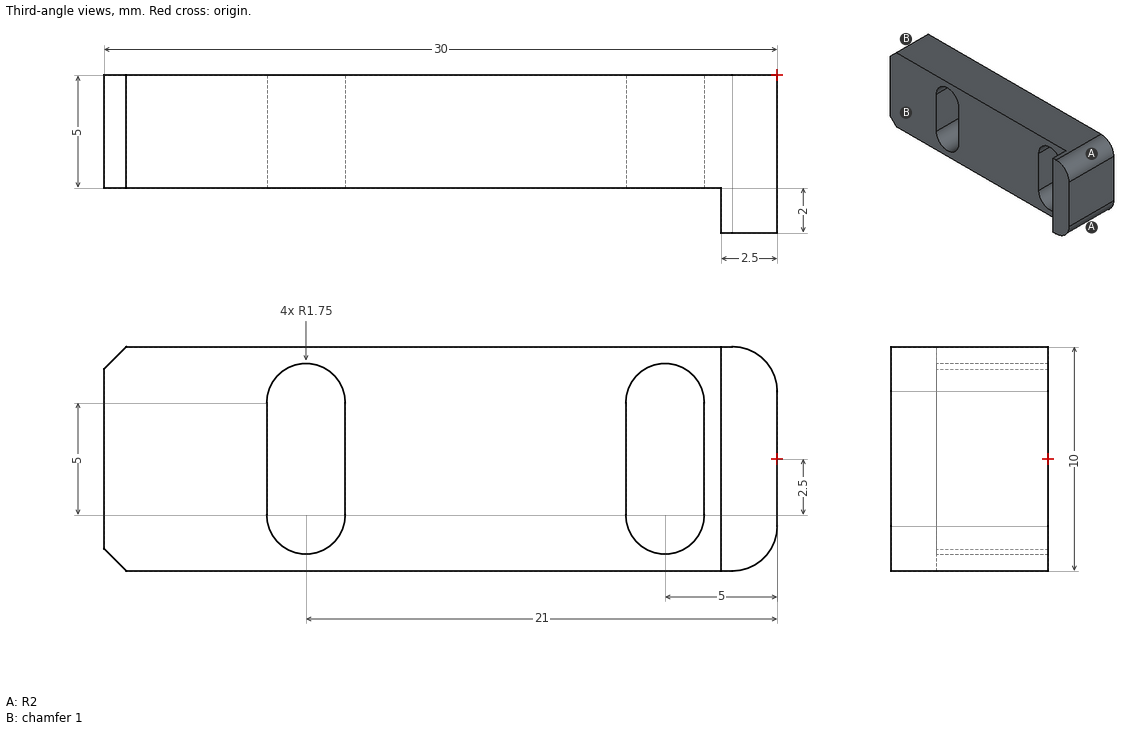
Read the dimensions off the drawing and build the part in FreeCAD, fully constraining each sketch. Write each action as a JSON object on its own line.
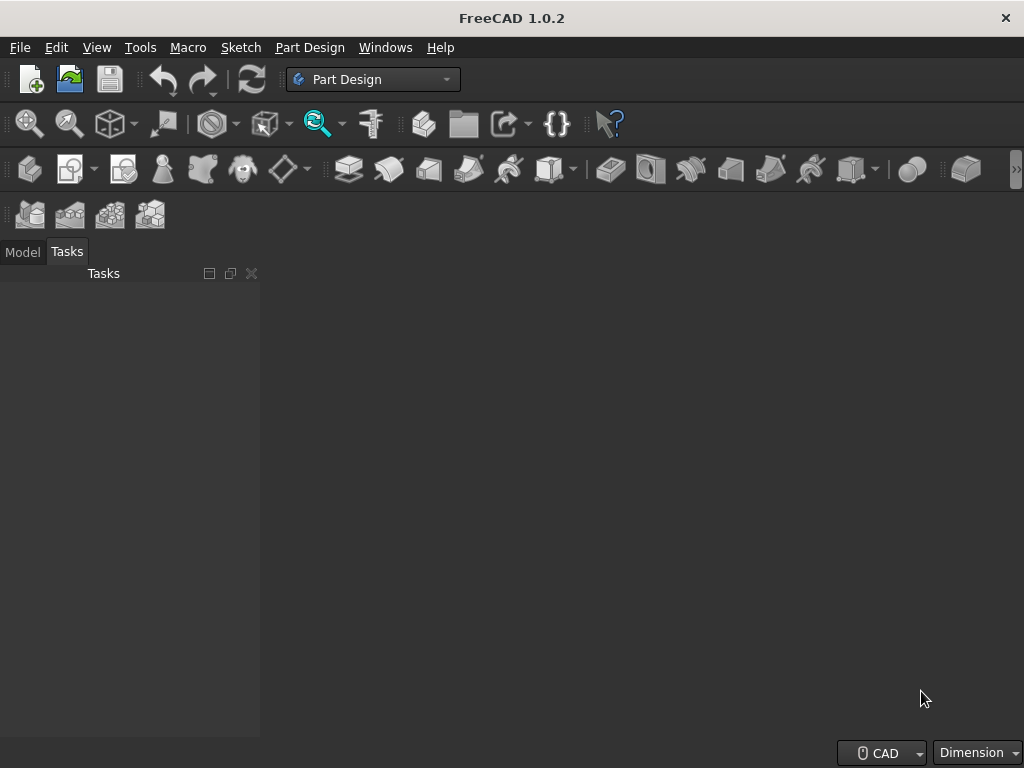
{"action": "left_click", "coordinate": [30, 80]}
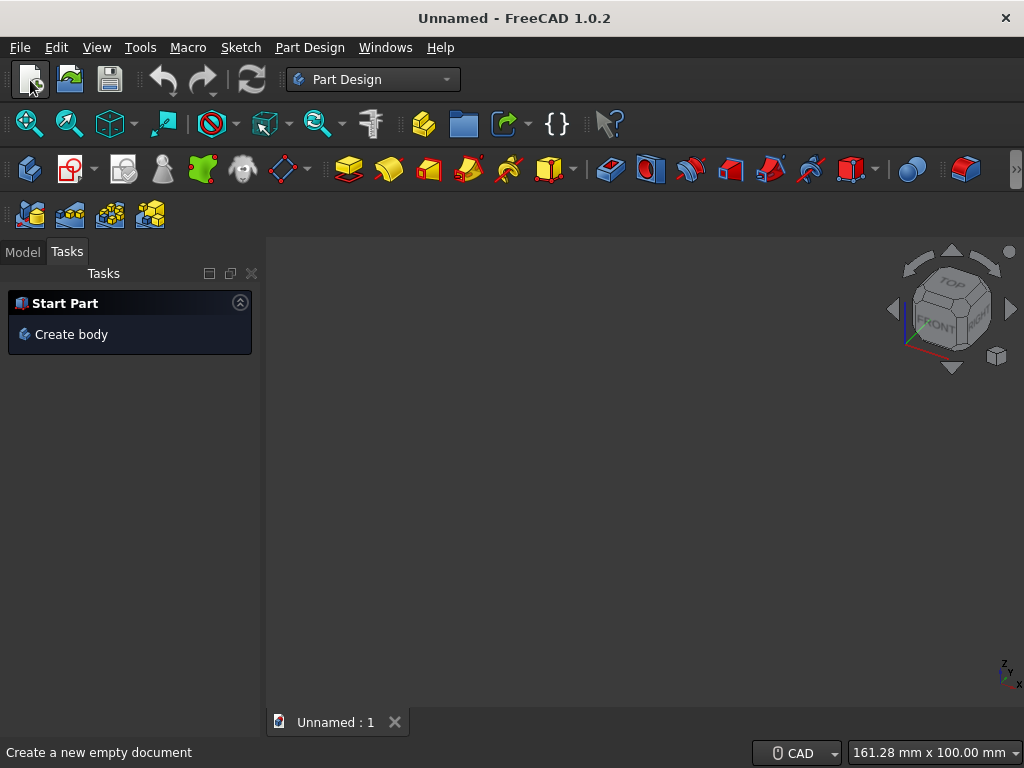
{"action": "left_click", "coordinate": [70, 170]}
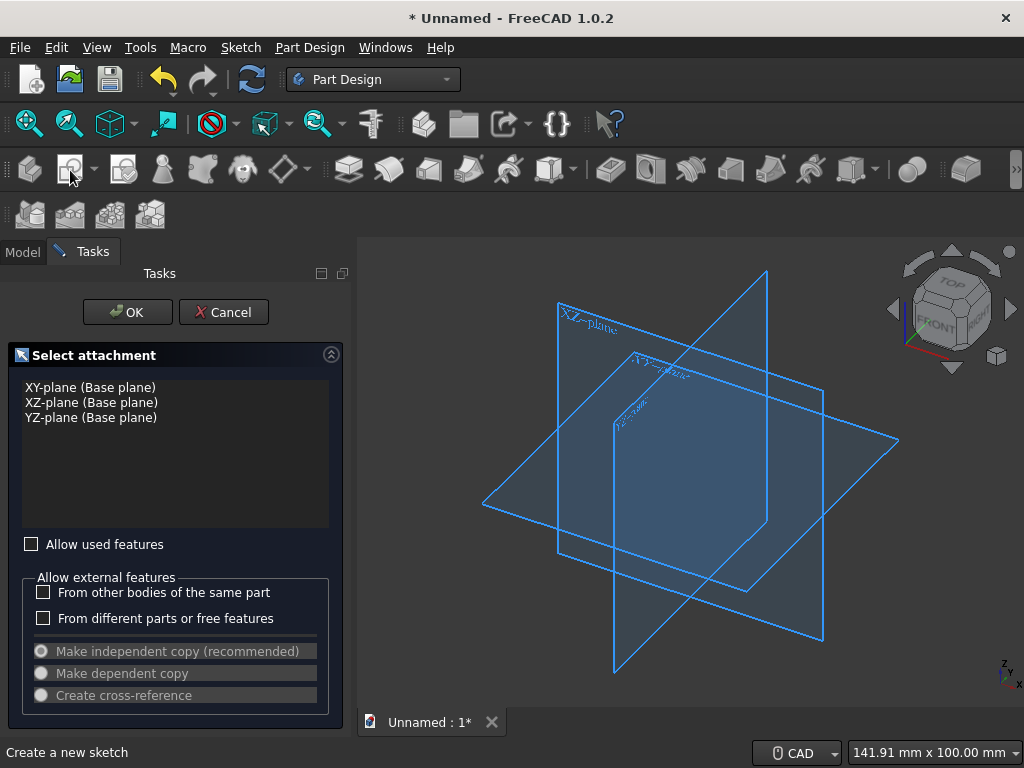
{"action": "left_click", "coordinate": [82, 388]}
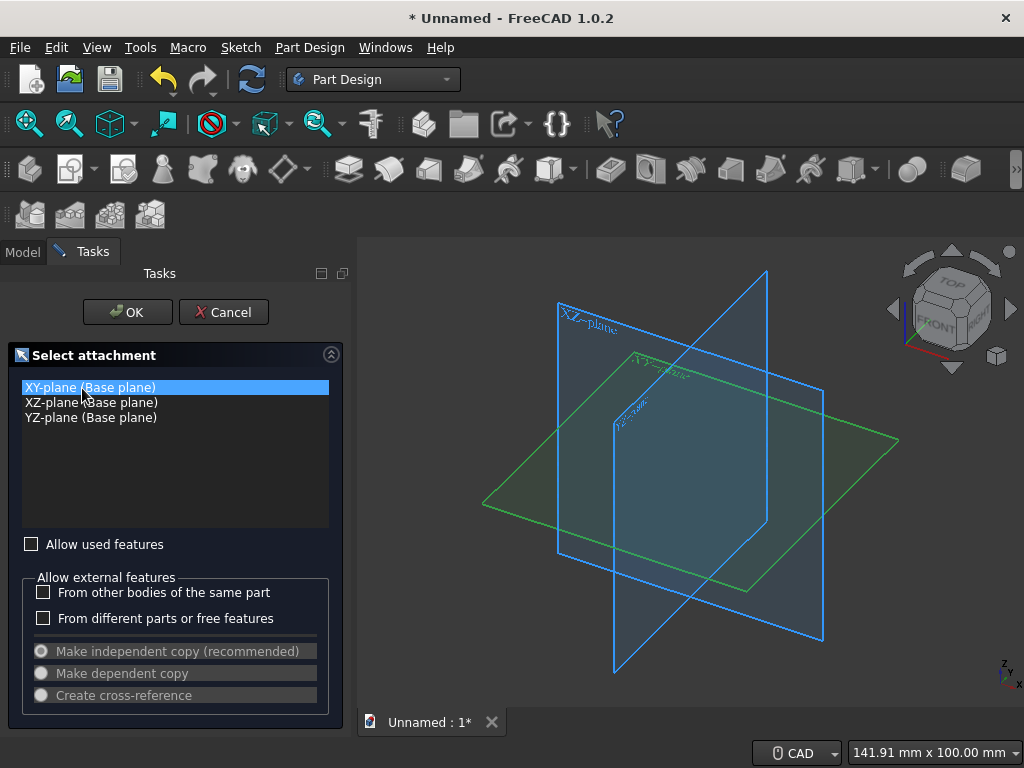
{"action": "left_click", "coordinate": [128, 312]}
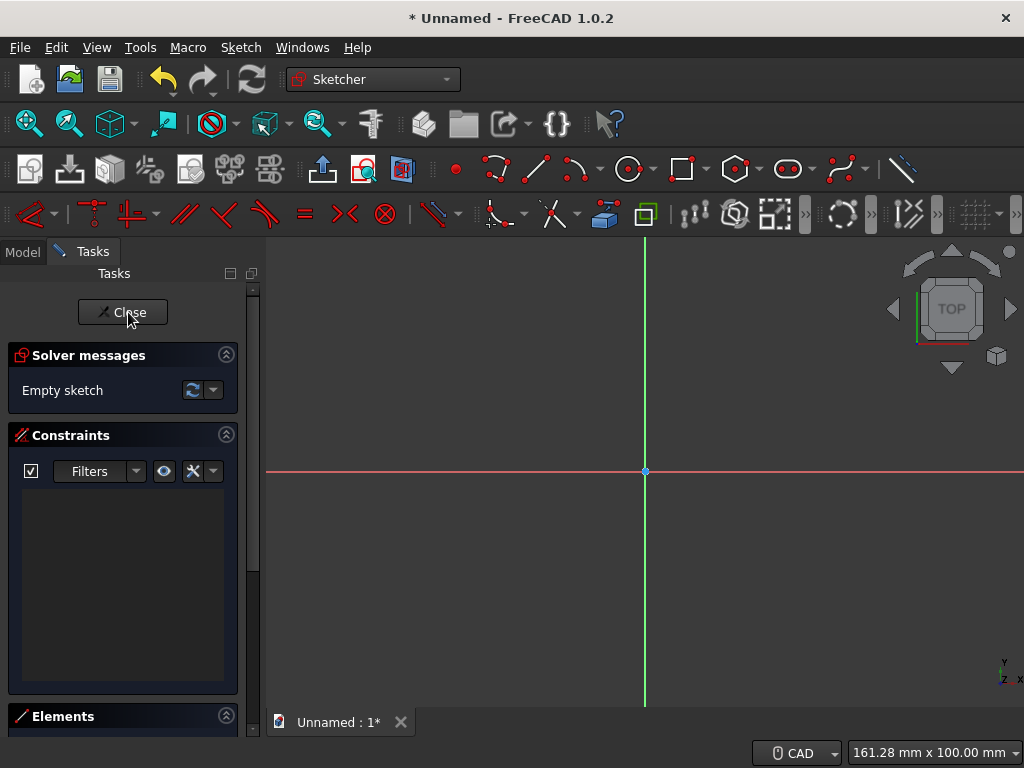
{"action": "scroll", "coordinate": [573, 498], "scroll_direction": "up", "scroll_amount": 5}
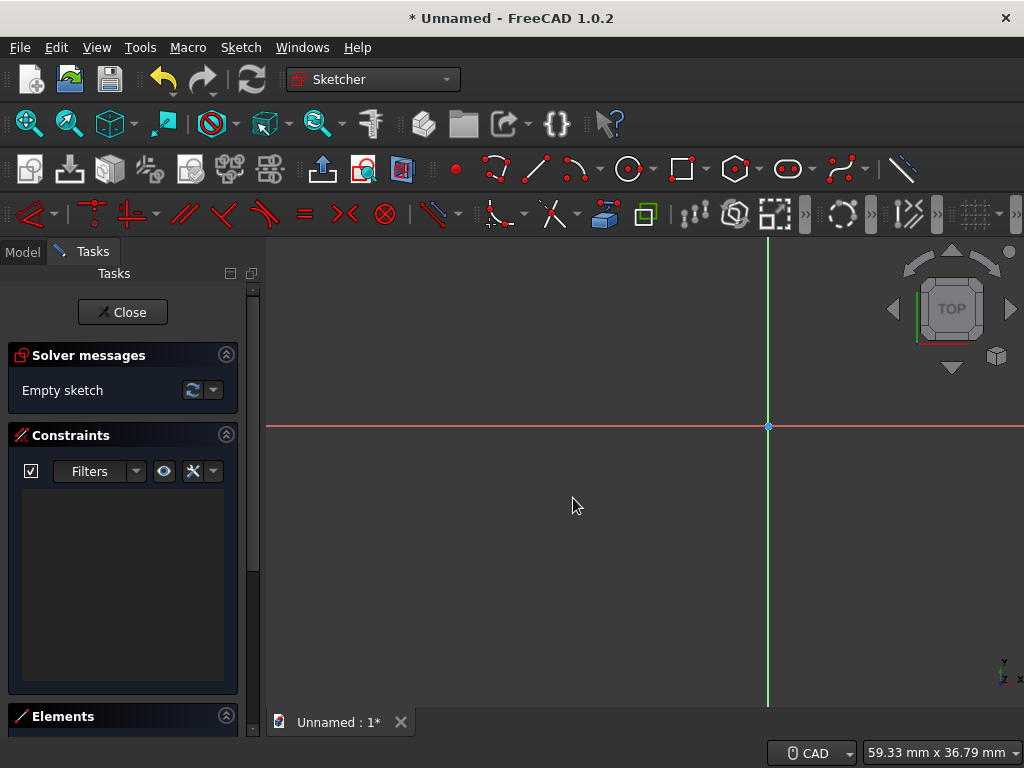
{"action": "left_click", "coordinate": [496, 170]}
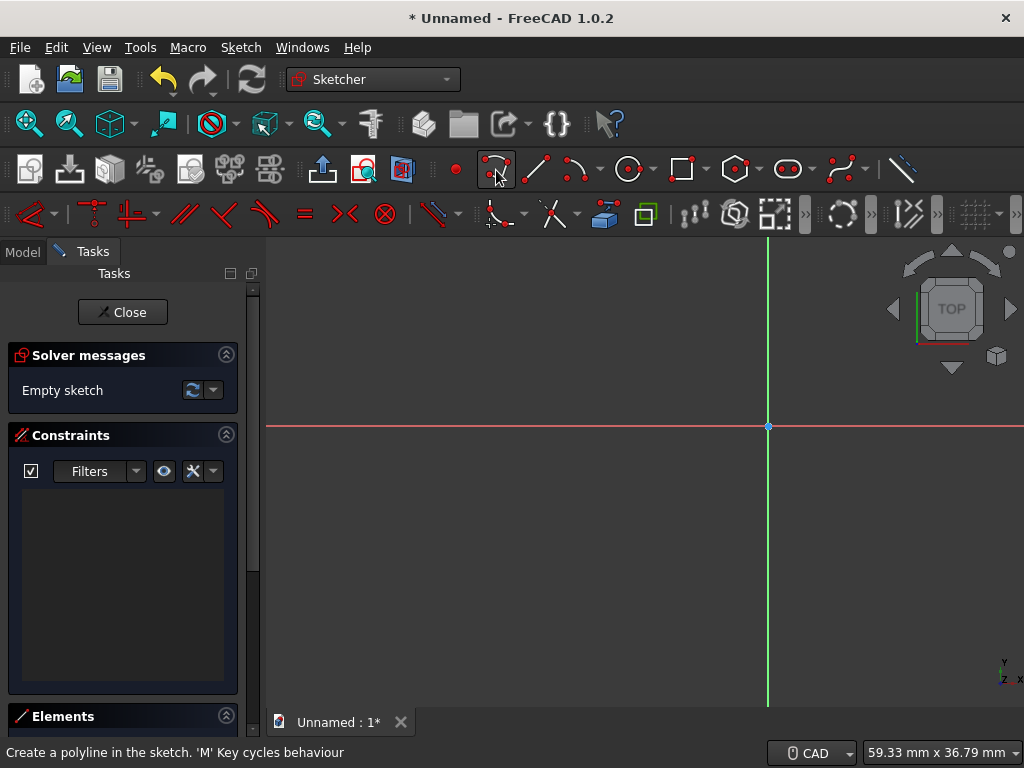
{"action": "left_click", "coordinate": [768, 426]}
{"action": "left_click", "coordinate": [385, 435]}
{"action": "left_click", "coordinate": [385, 490]}
{"action": "left_click", "coordinate": [736, 490]}
{"action": "left_click", "coordinate": [736, 516]}
{"action": "left_click", "coordinate": [759, 516]}
{"action": "left_click", "coordinate": [768, 426]}
{"action": "key", "text": "Escape"}
{"action": "key", "text": "Escape"}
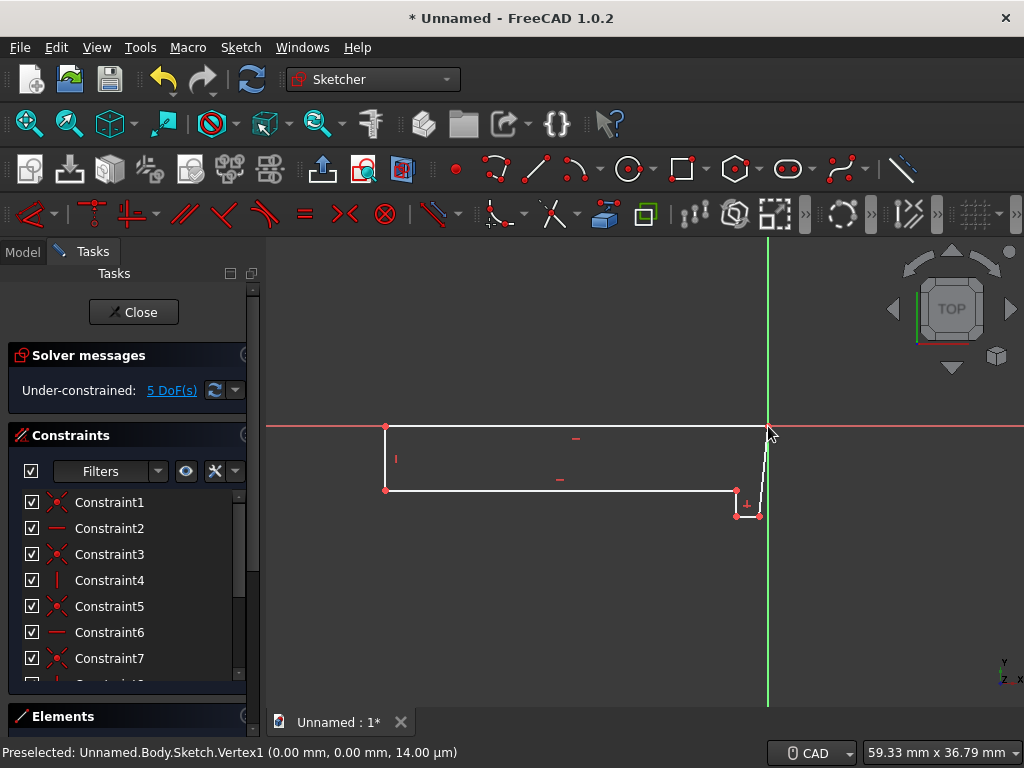
{"action": "left_click", "coordinate": [765, 454]}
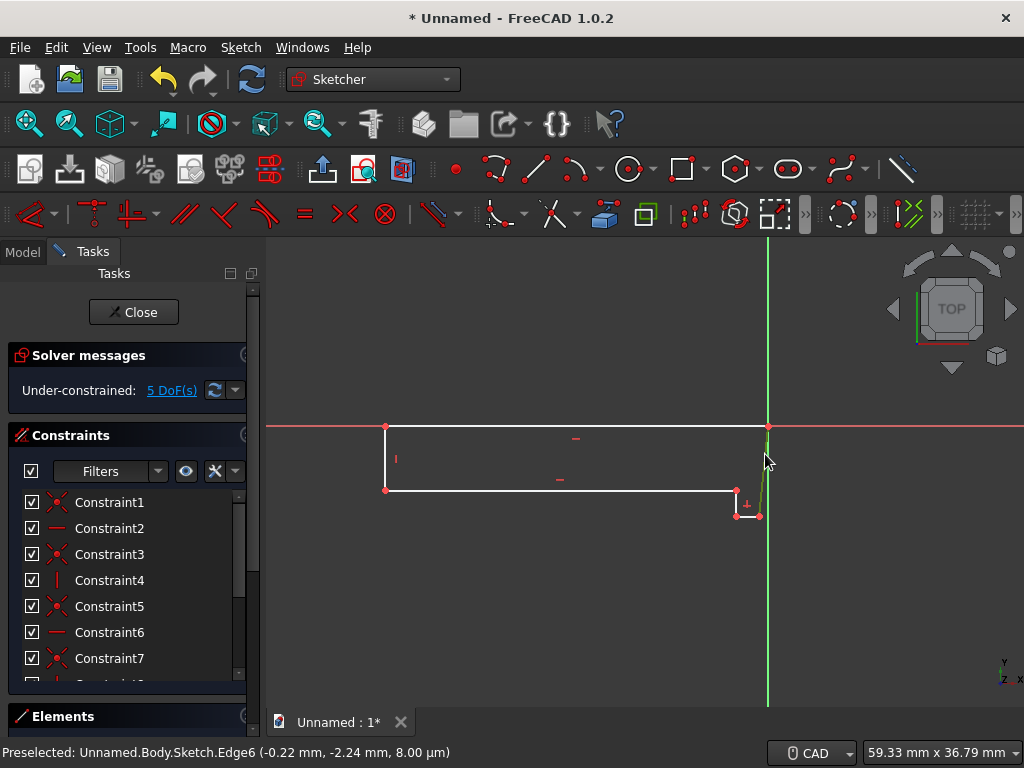
{"action": "left_click", "coordinate": [158, 214]}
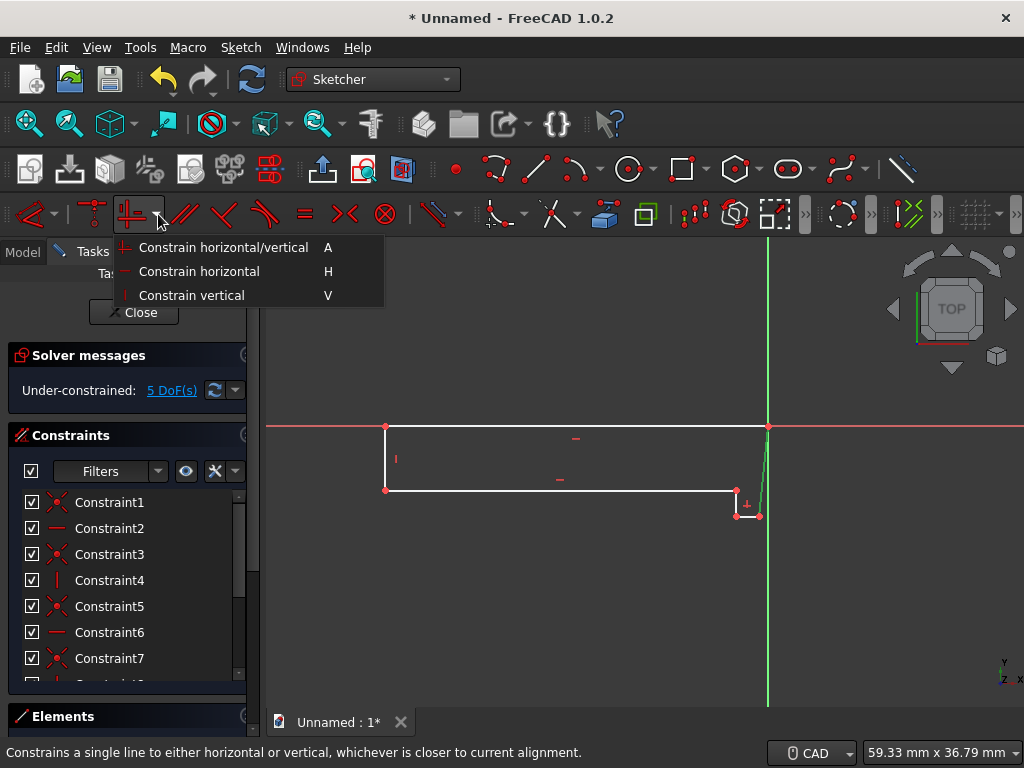
{"action": "left_click", "coordinate": [249, 295]}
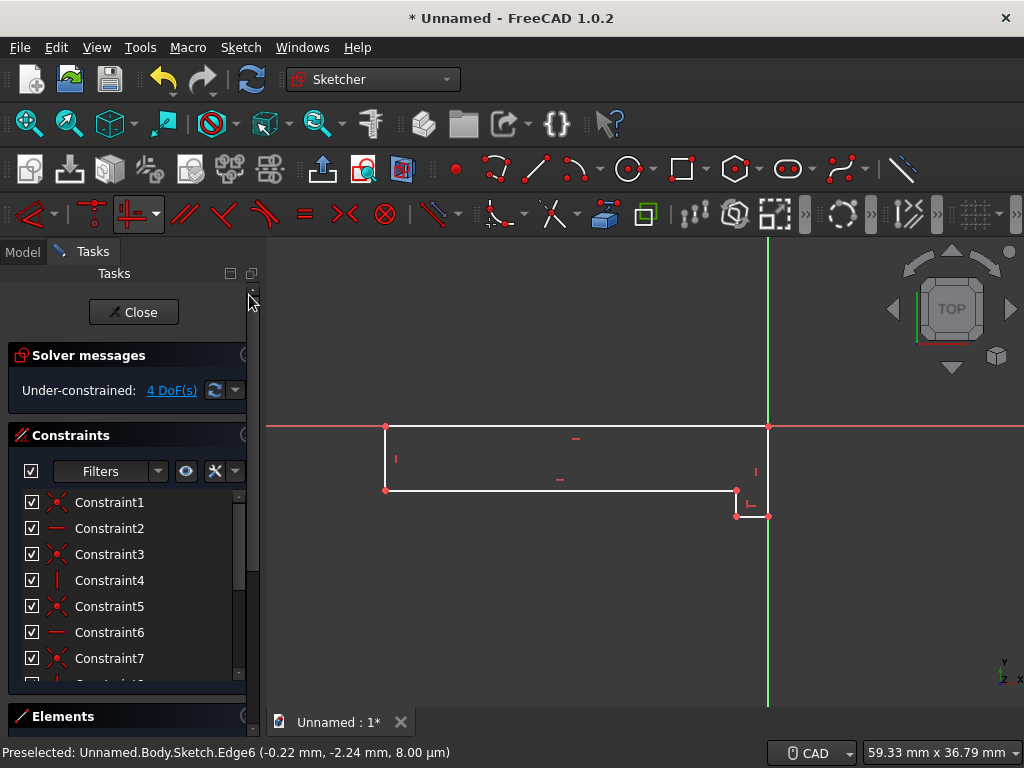
{"action": "left_click", "coordinate": [385, 446]}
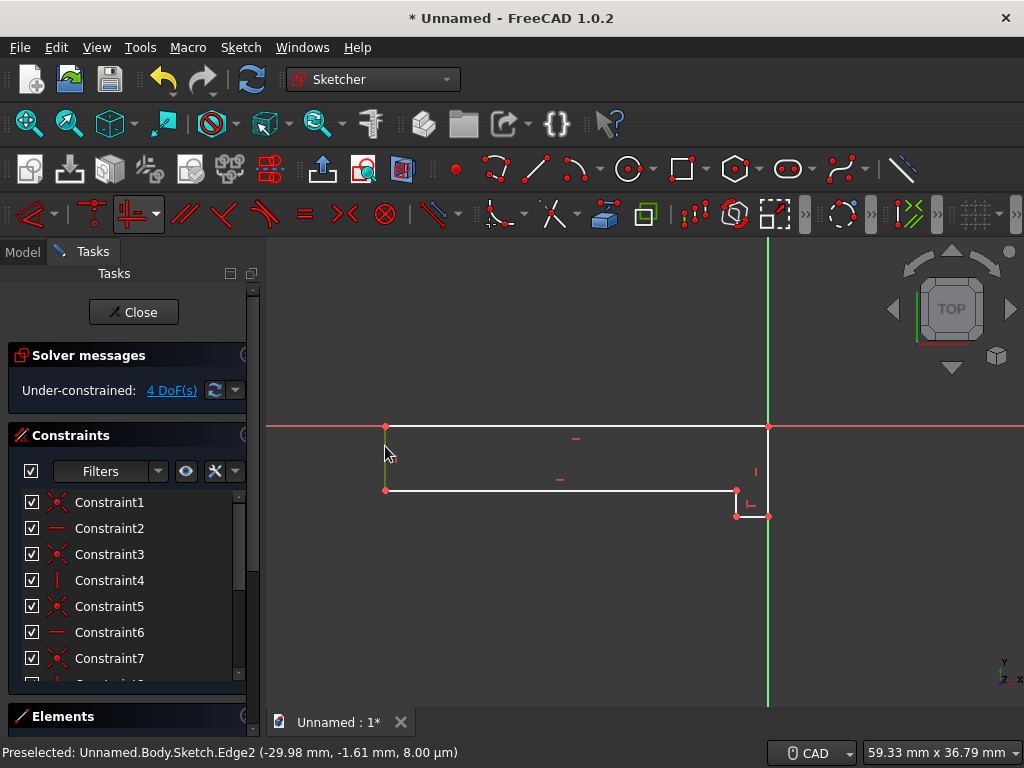
{"action": "key", "text": "i"}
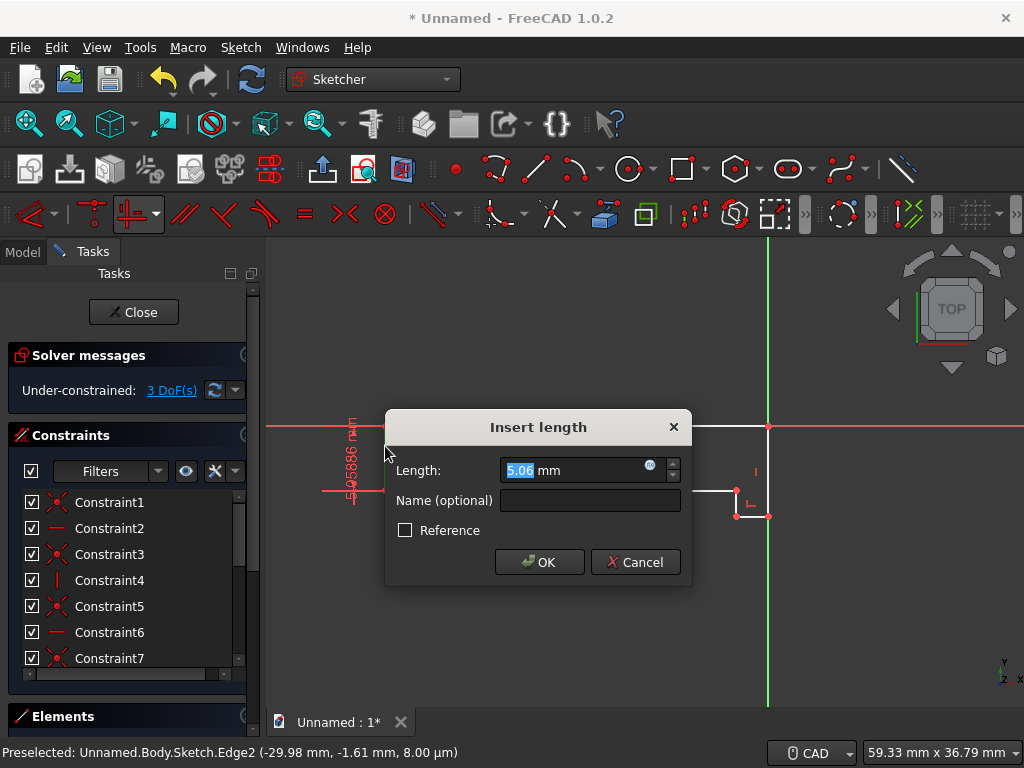
{"action": "type", "text": "5"}
{"action": "key", "text": "Return"}